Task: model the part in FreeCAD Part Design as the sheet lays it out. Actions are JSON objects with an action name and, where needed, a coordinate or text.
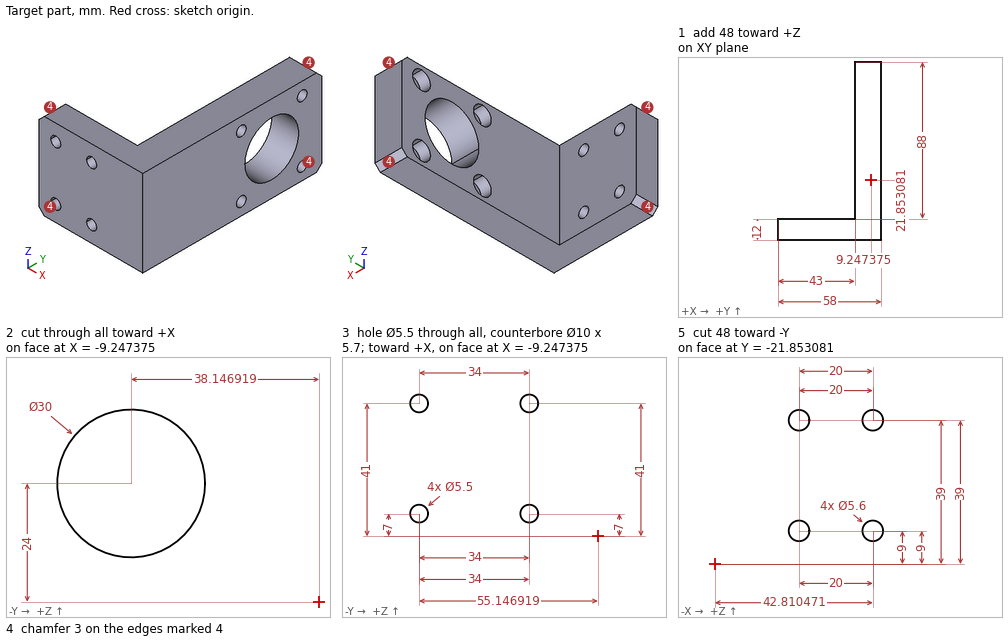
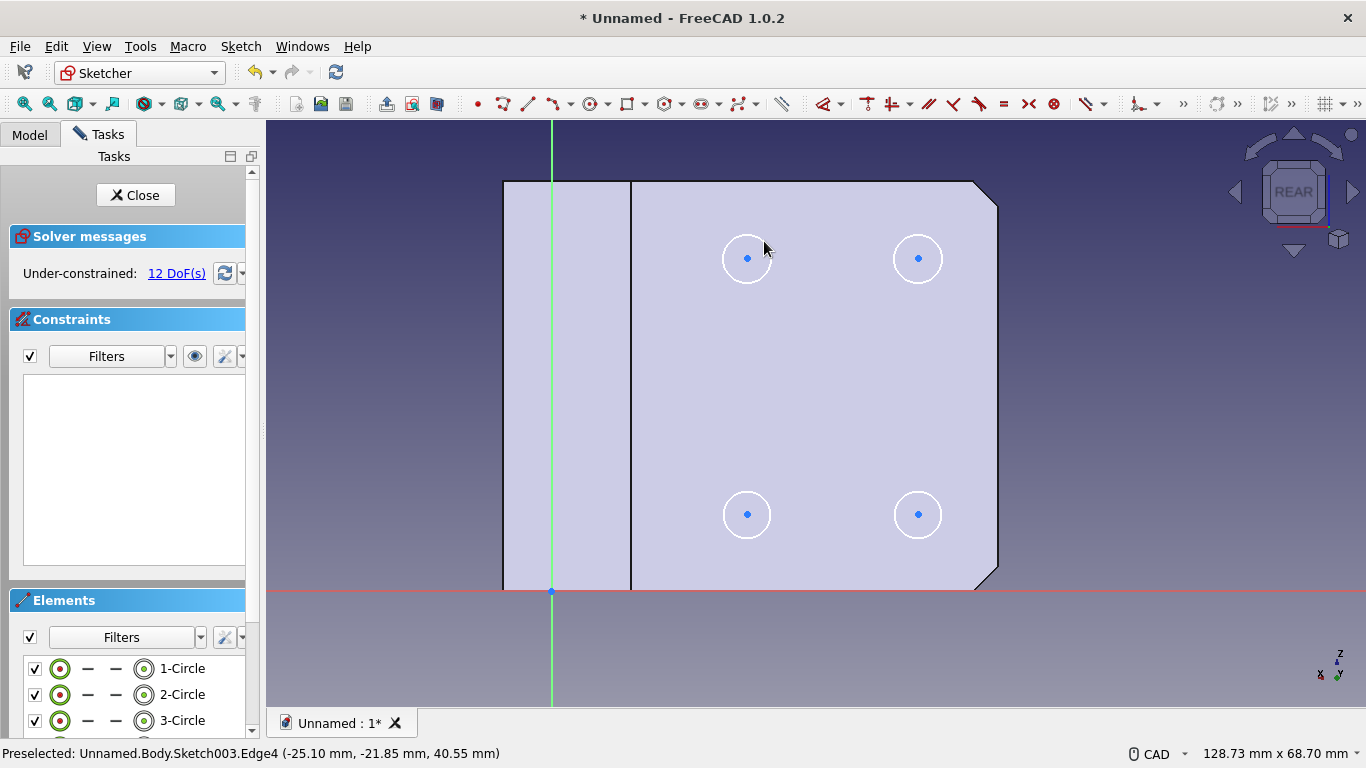
{"action": "left_click", "coordinate": [934, 498]}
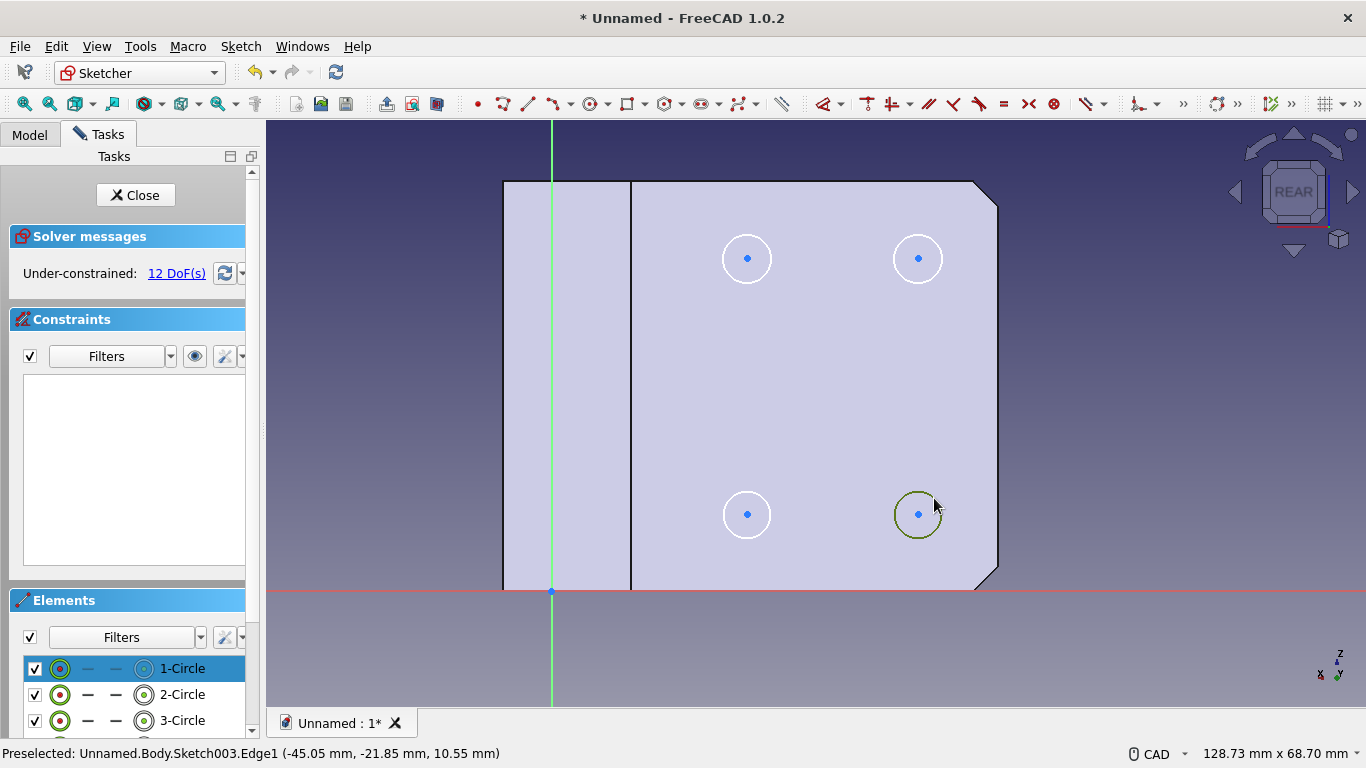
{"action": "left_click", "coordinate": [763, 498]}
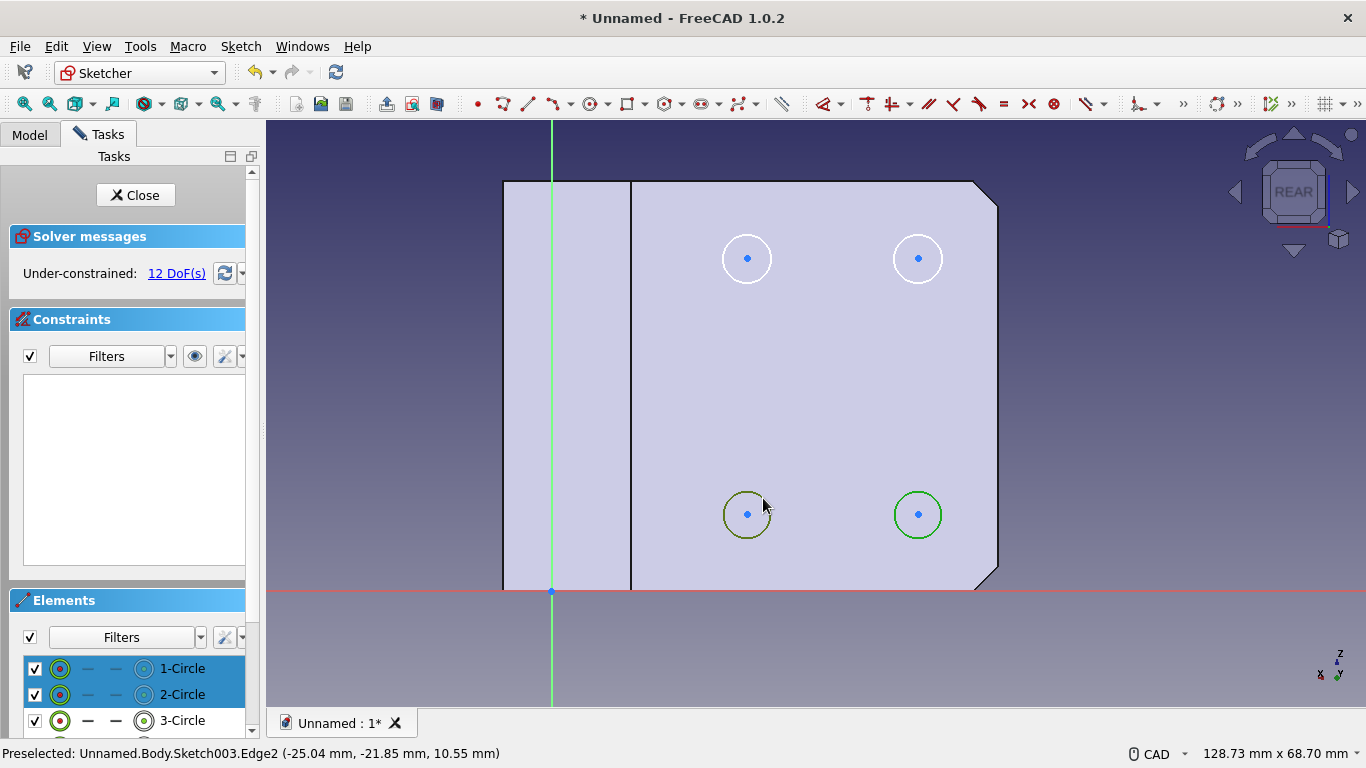
{"action": "left_click", "coordinate": [935, 242]}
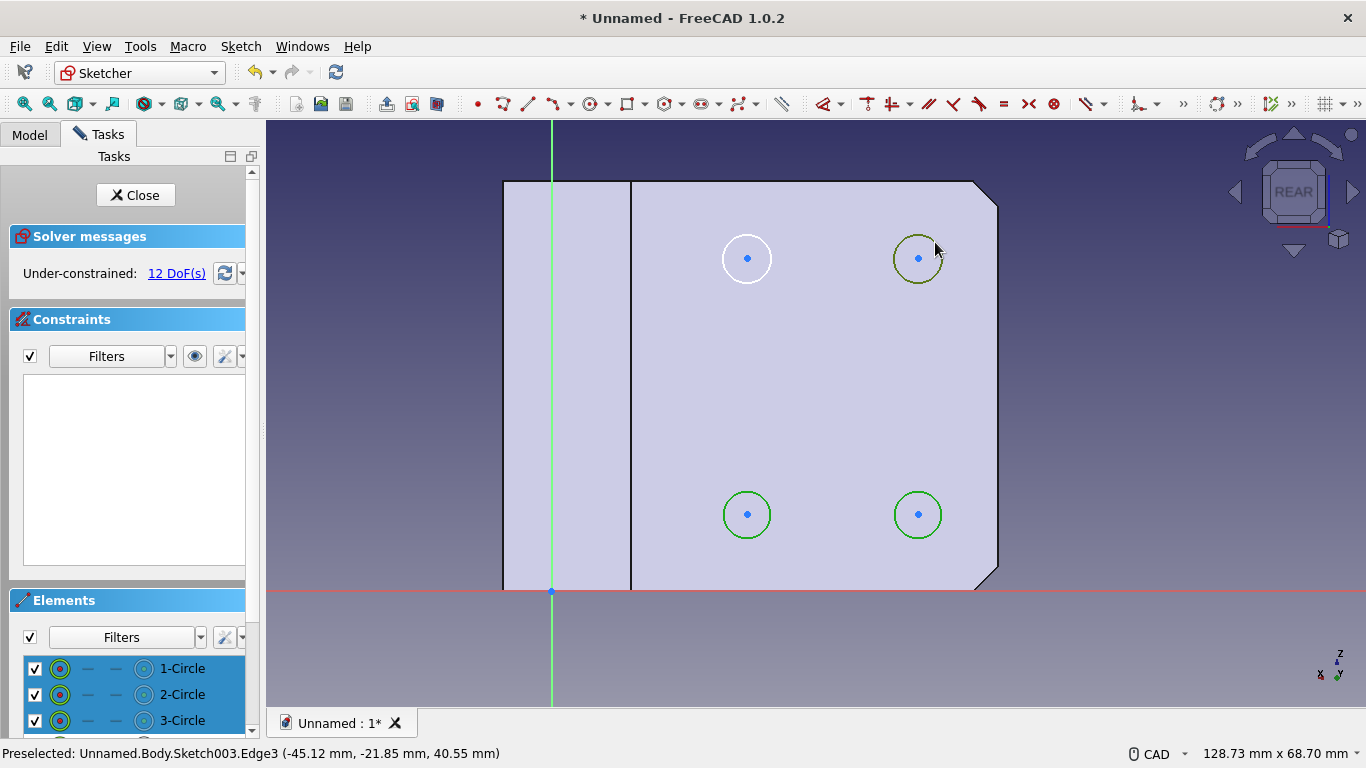
{"action": "left_click", "coordinate": [764, 242]}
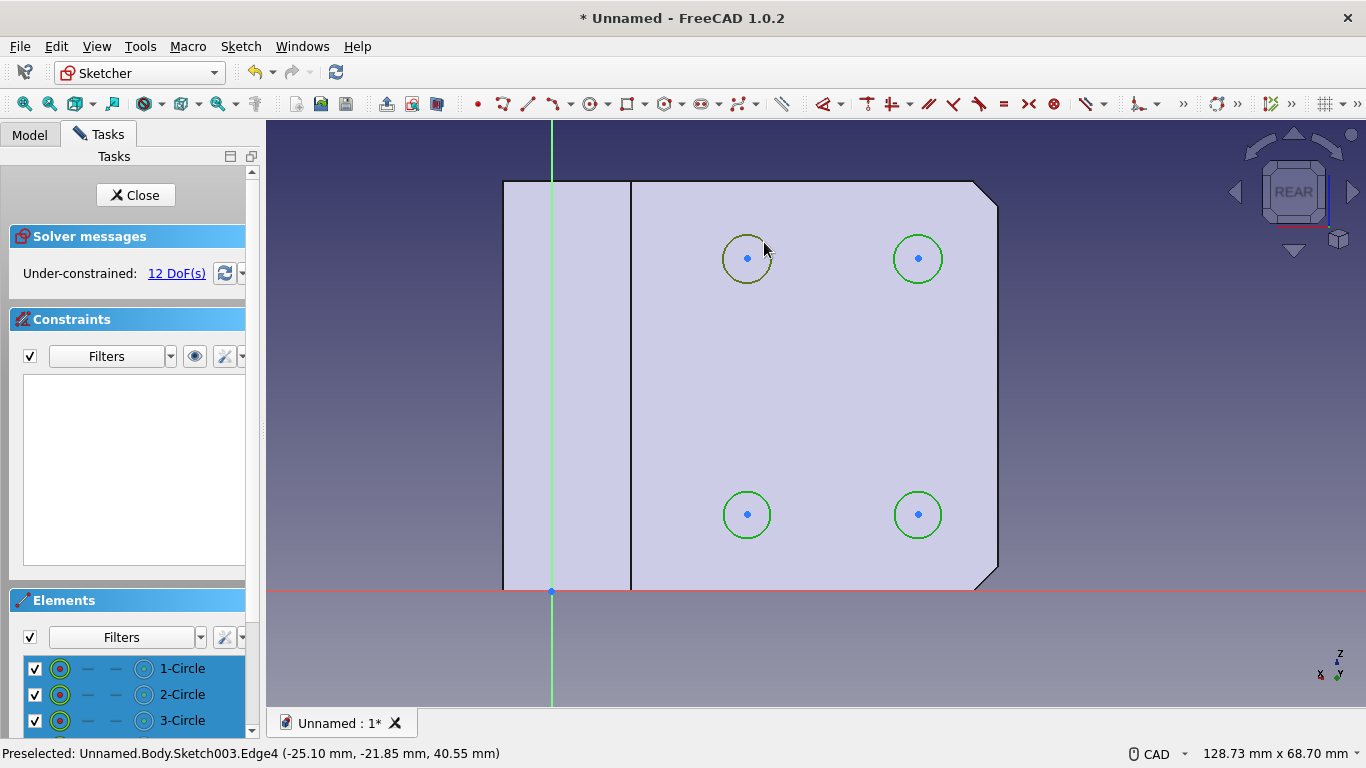
{"action": "left_click", "coordinate": [1004, 104]}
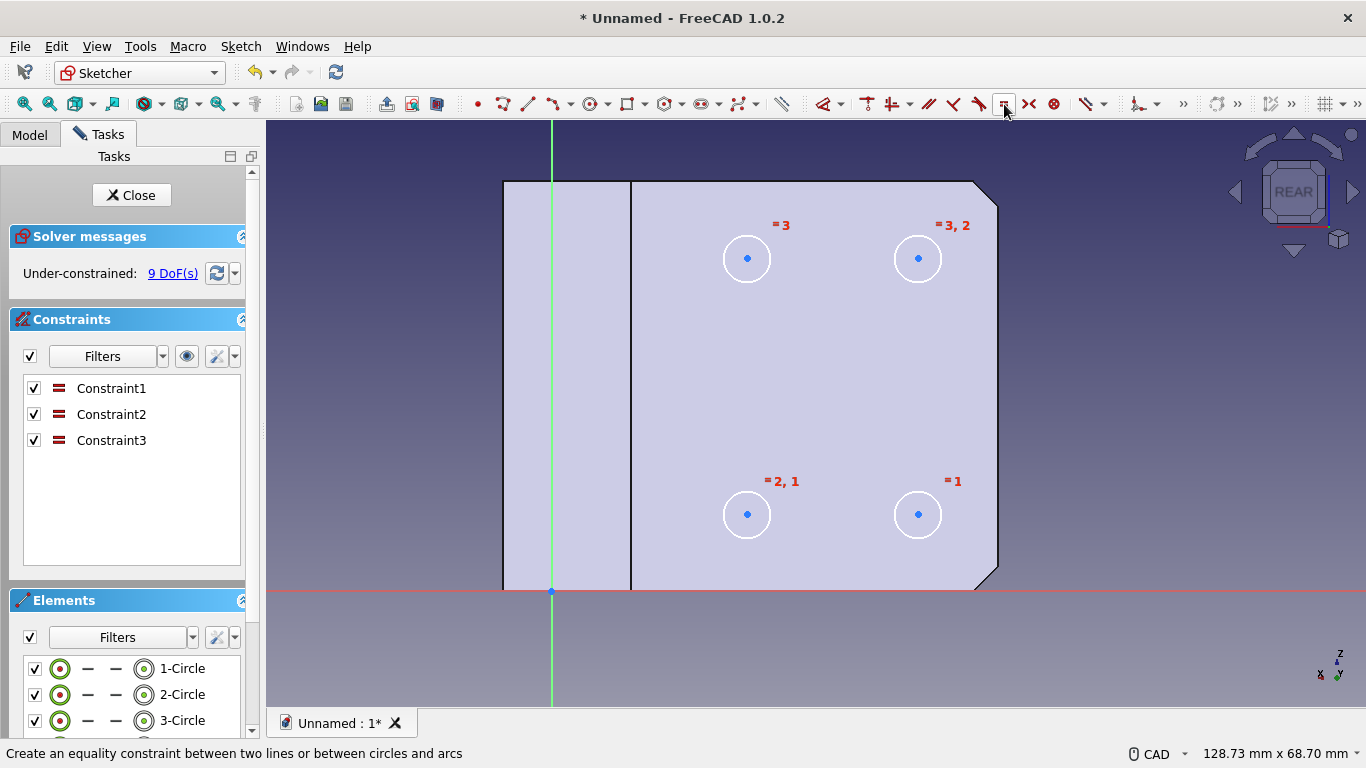
{"action": "left_click", "coordinate": [822, 104]}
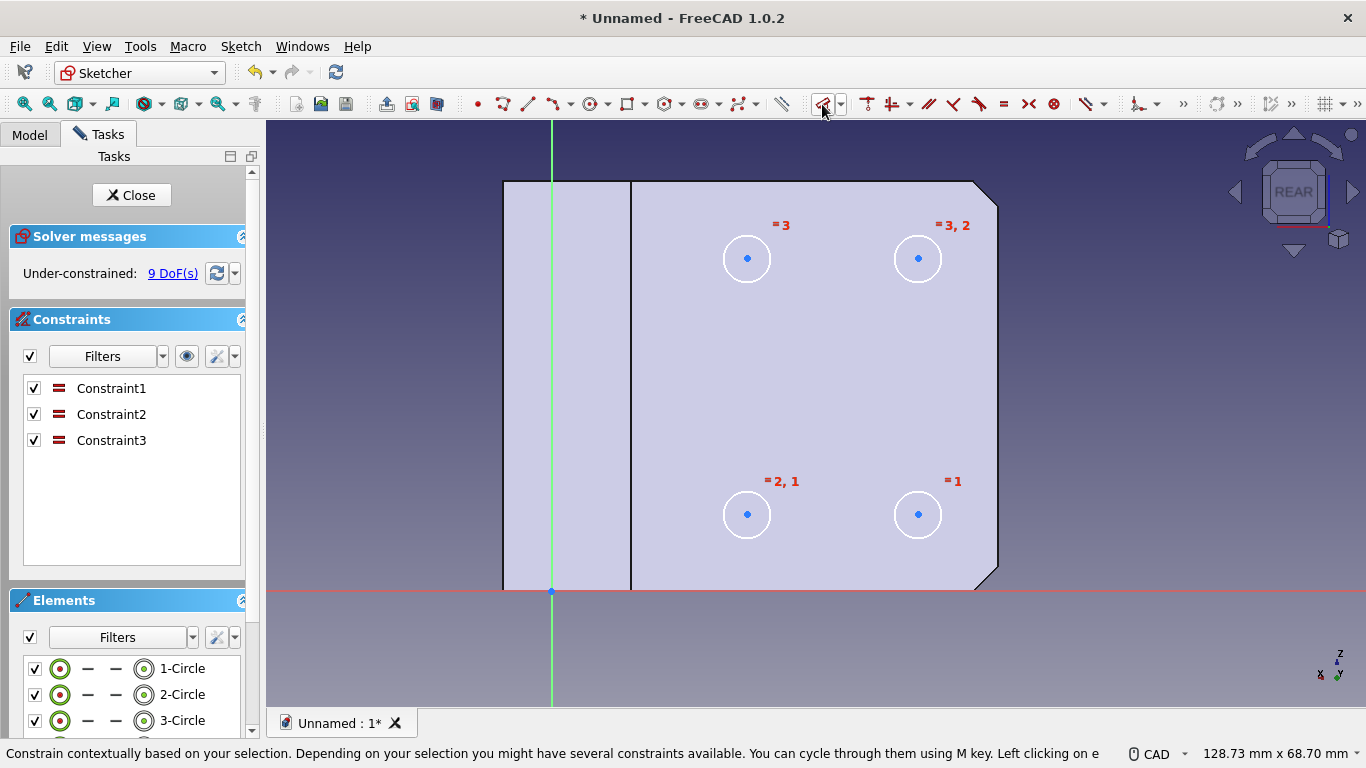
{"action": "left_click", "coordinate": [934, 498]}
{"action": "left_click", "coordinate": [956, 475]}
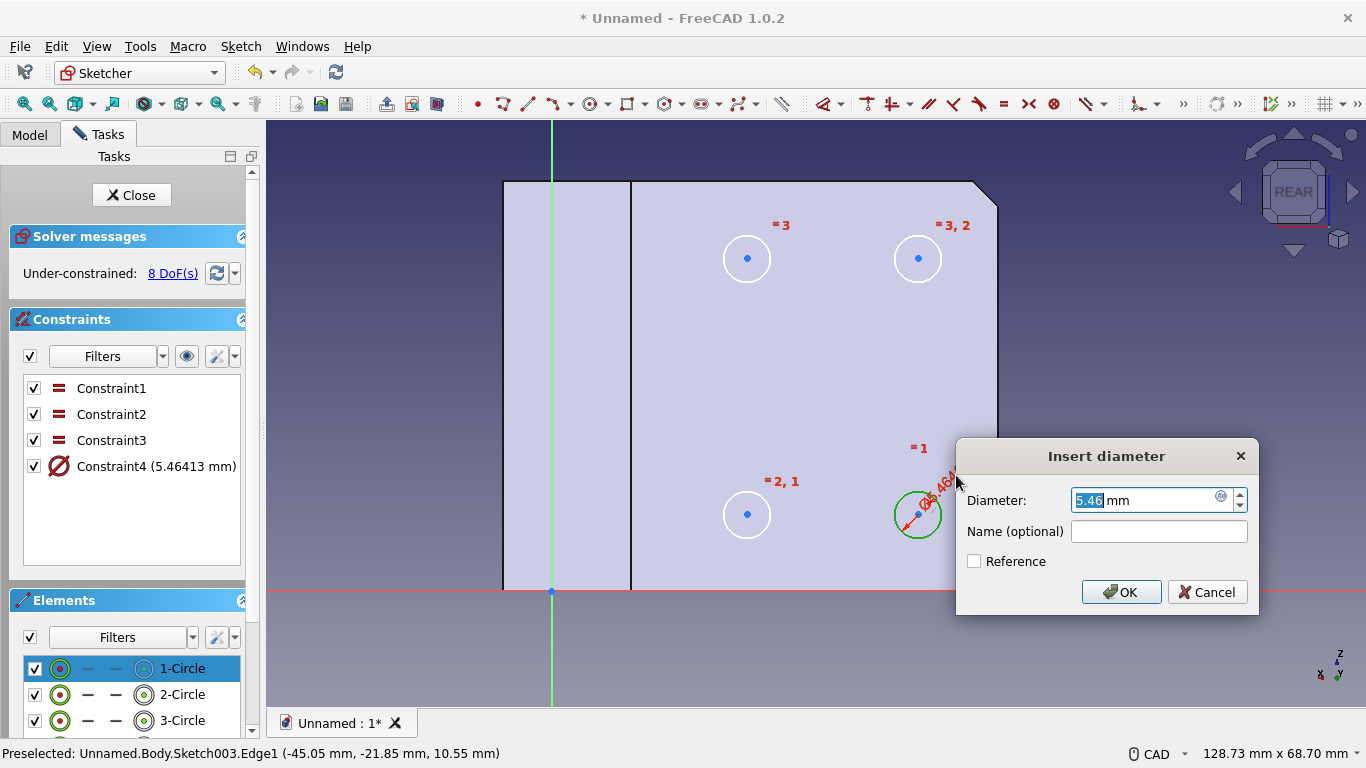
{"action": "type", "text": "5.6"}
{"action": "key", "text": "Return"}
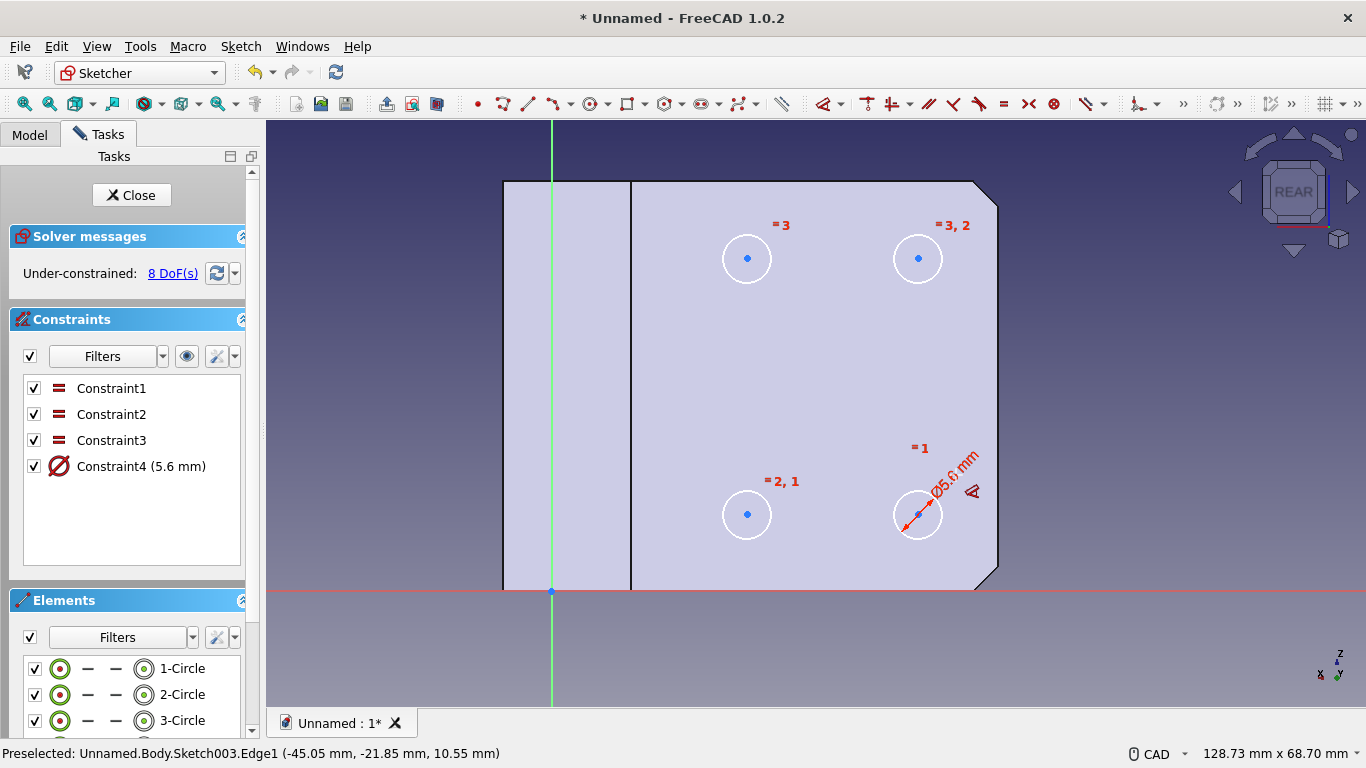
{"action": "left_click", "coordinate": [918, 515]}
{"action": "left_click", "coordinate": [518, 553]}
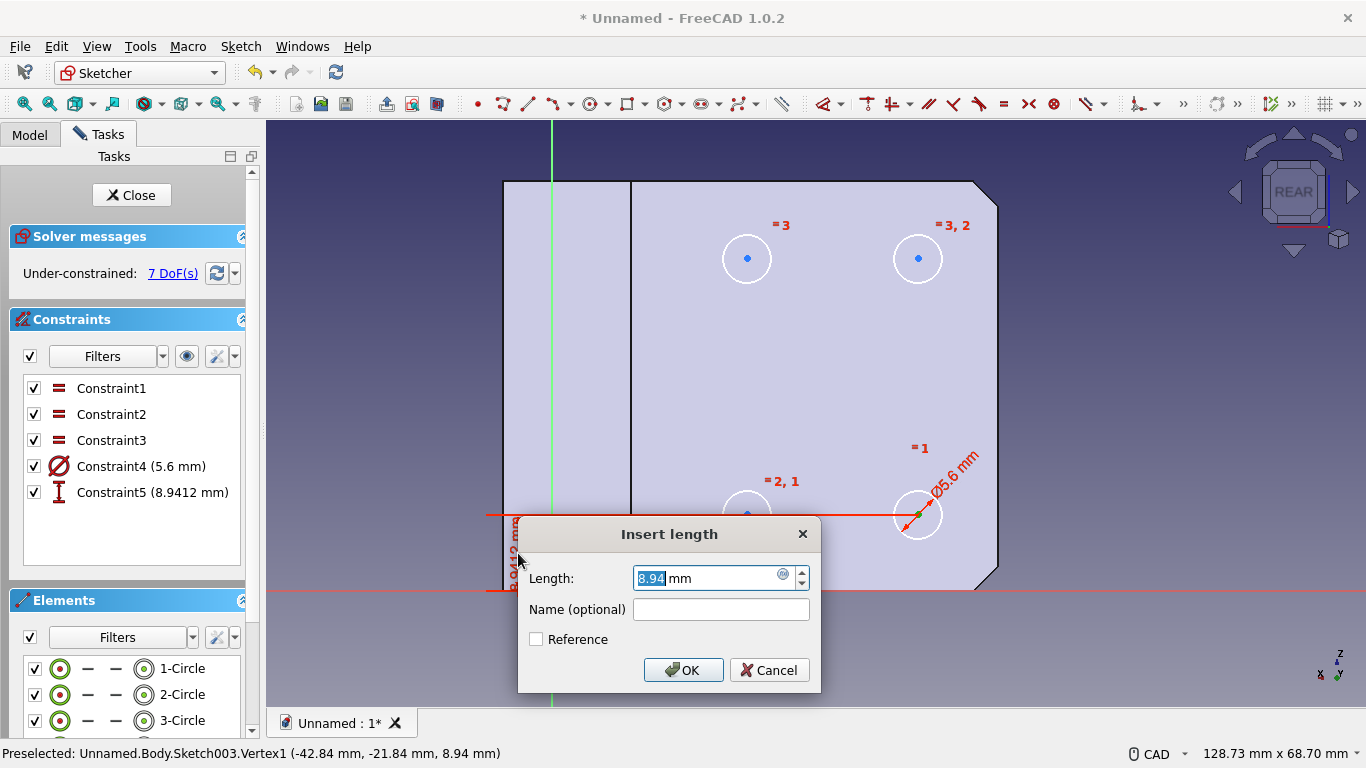
{"action": "type", "text": "9"}
{"action": "key", "text": "Return"}